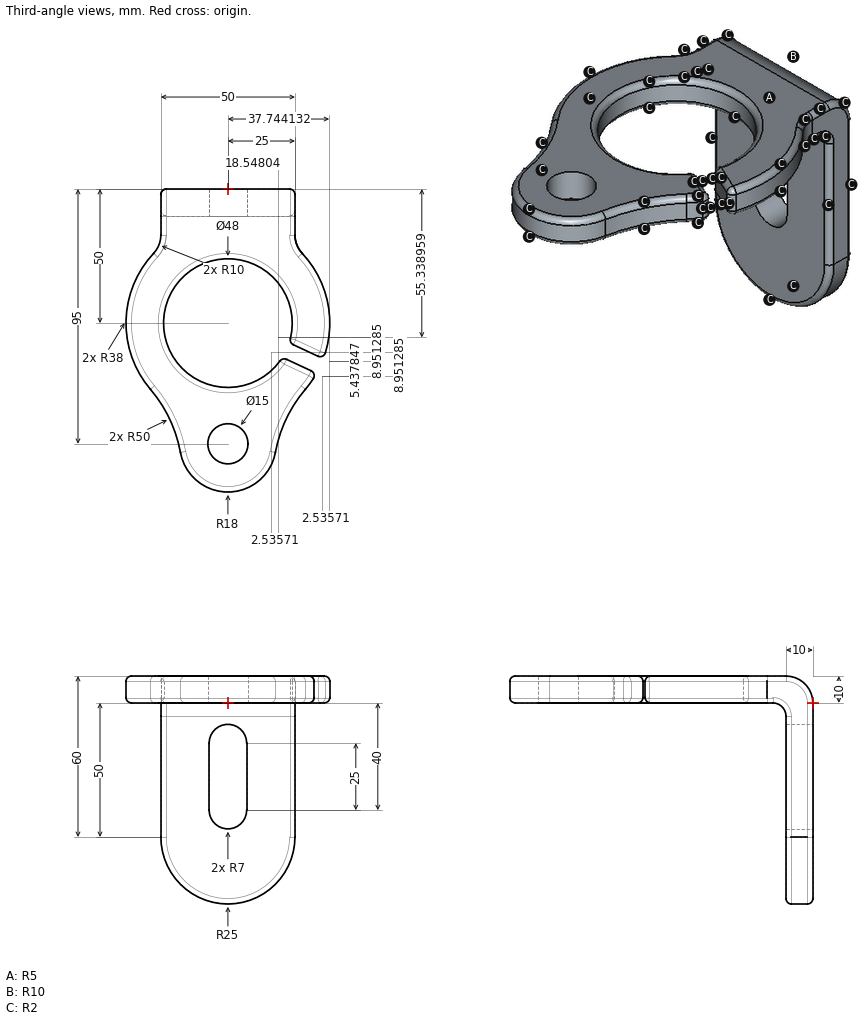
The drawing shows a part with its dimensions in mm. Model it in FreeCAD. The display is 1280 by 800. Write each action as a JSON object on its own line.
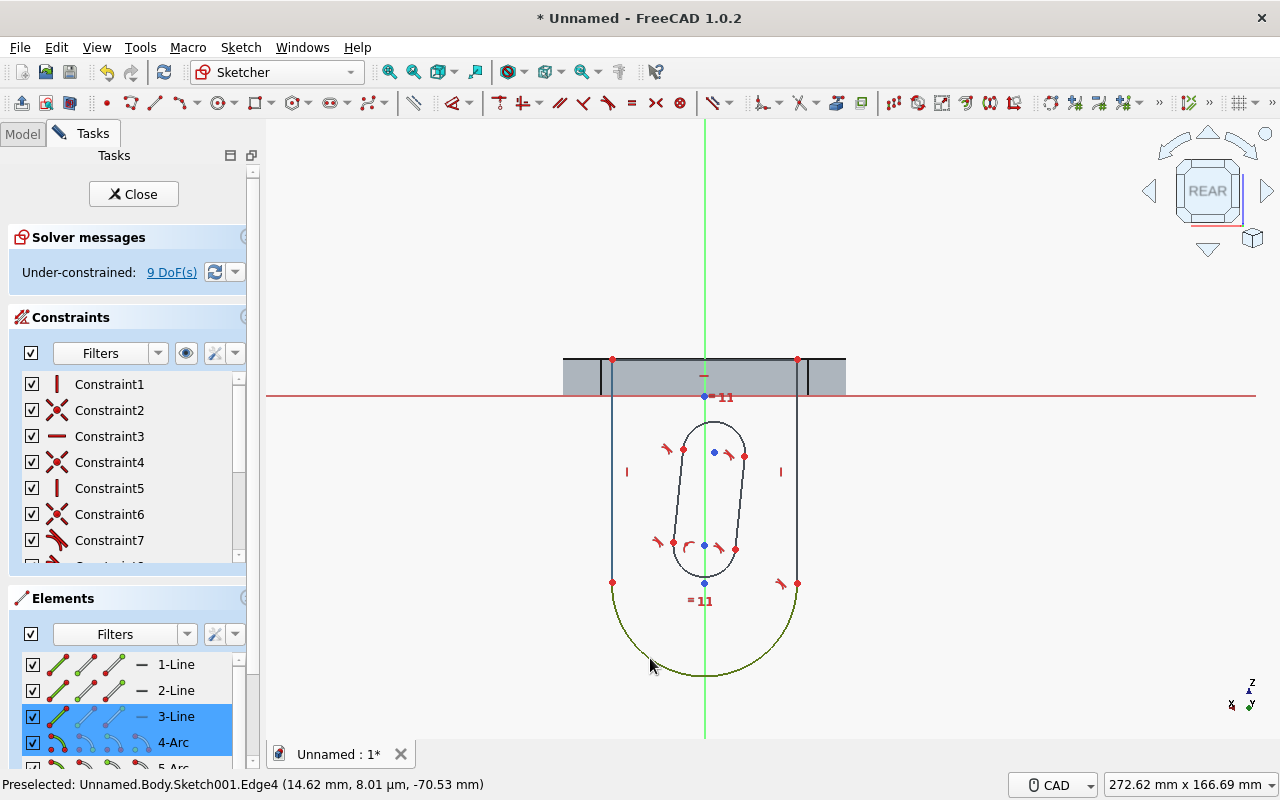
{"action": "left_click", "coordinate": [608, 104]}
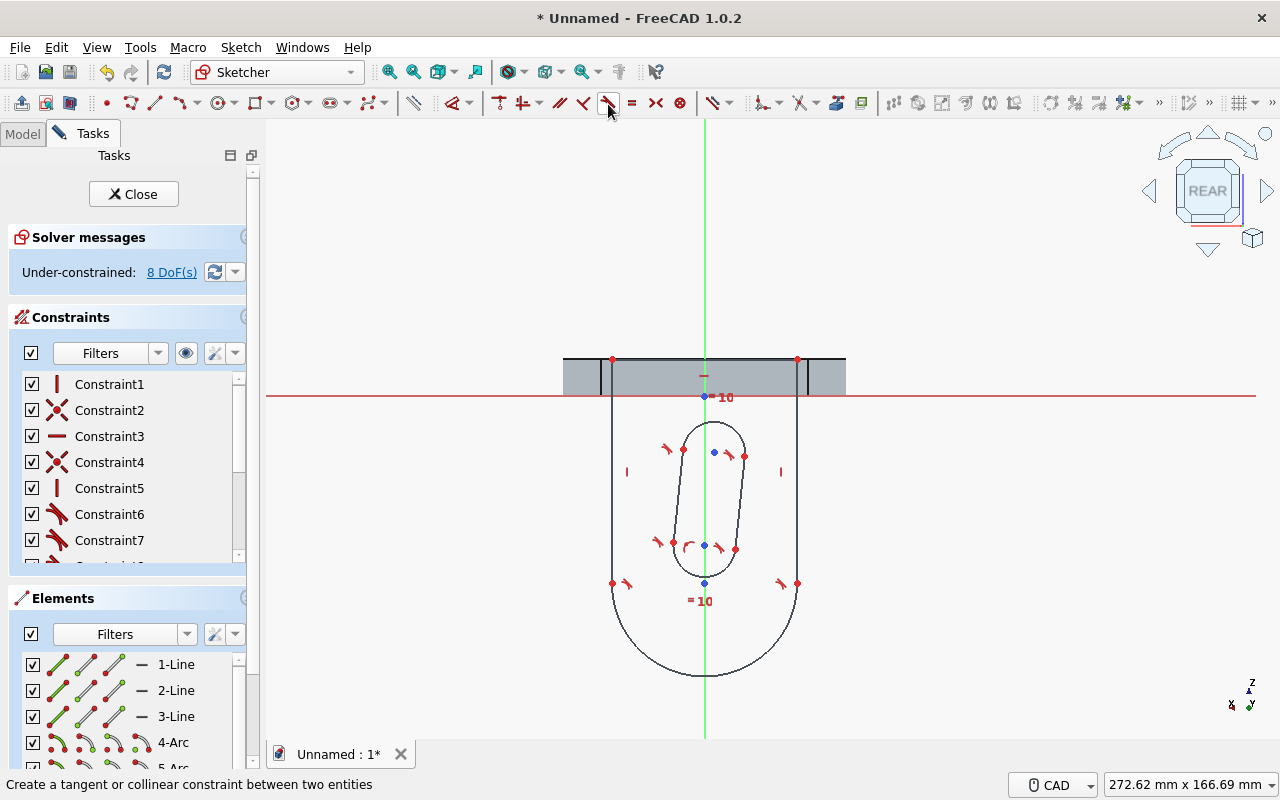
{"action": "left_click", "coordinate": [676, 515]}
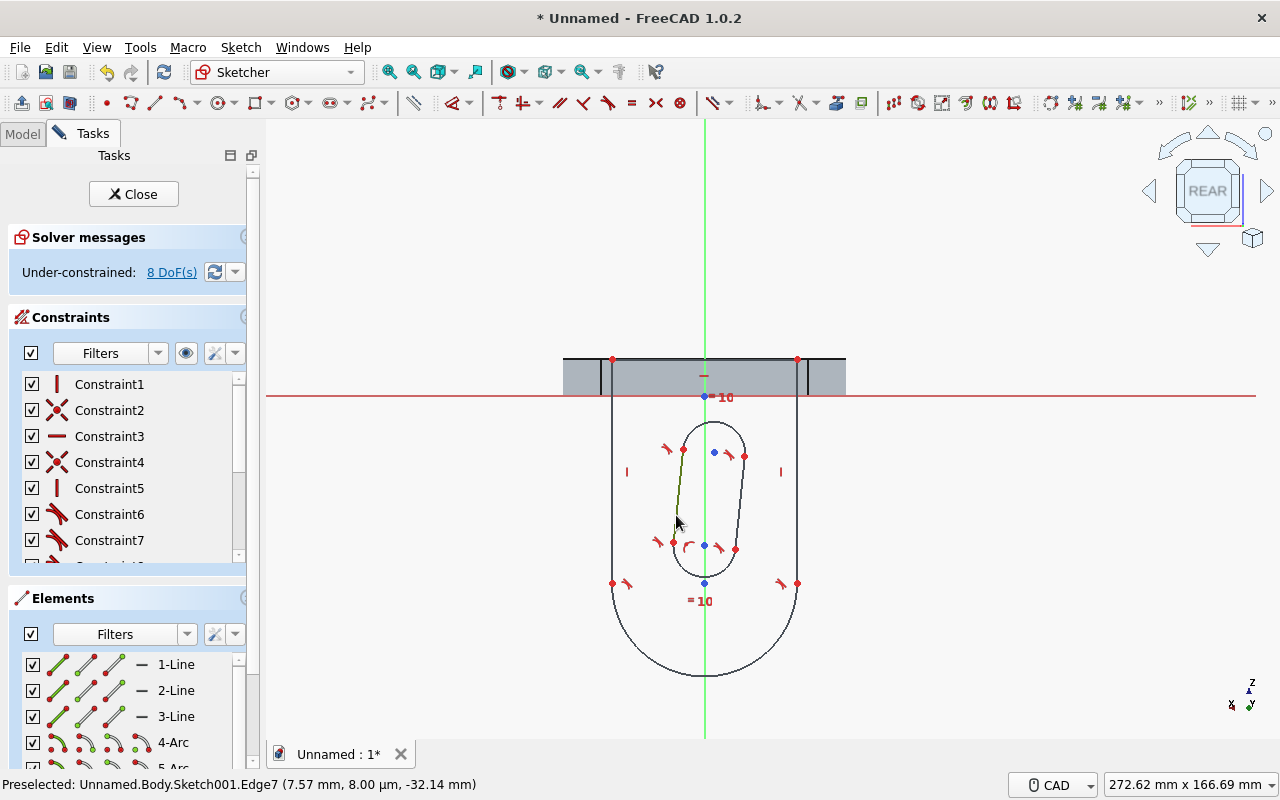
{"action": "key", "text": "v"}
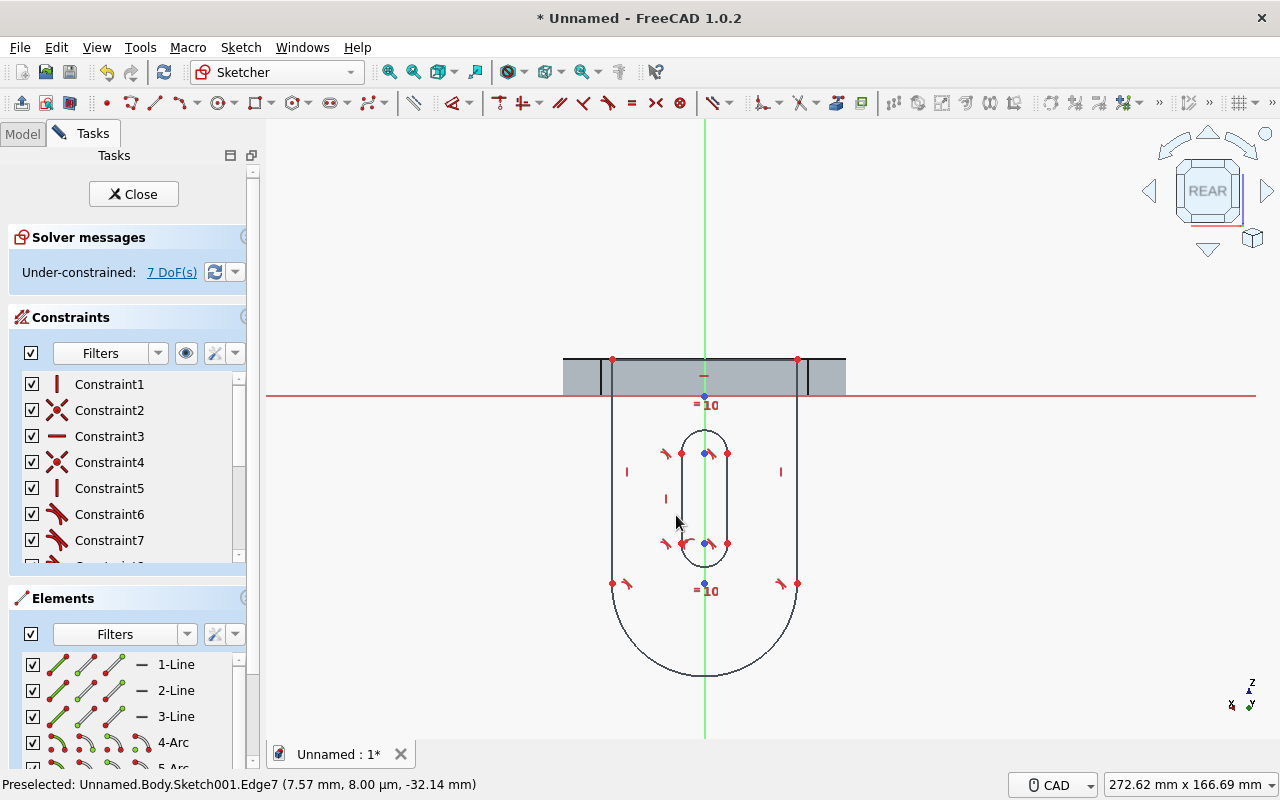
{"action": "left_click", "coordinate": [705, 584]}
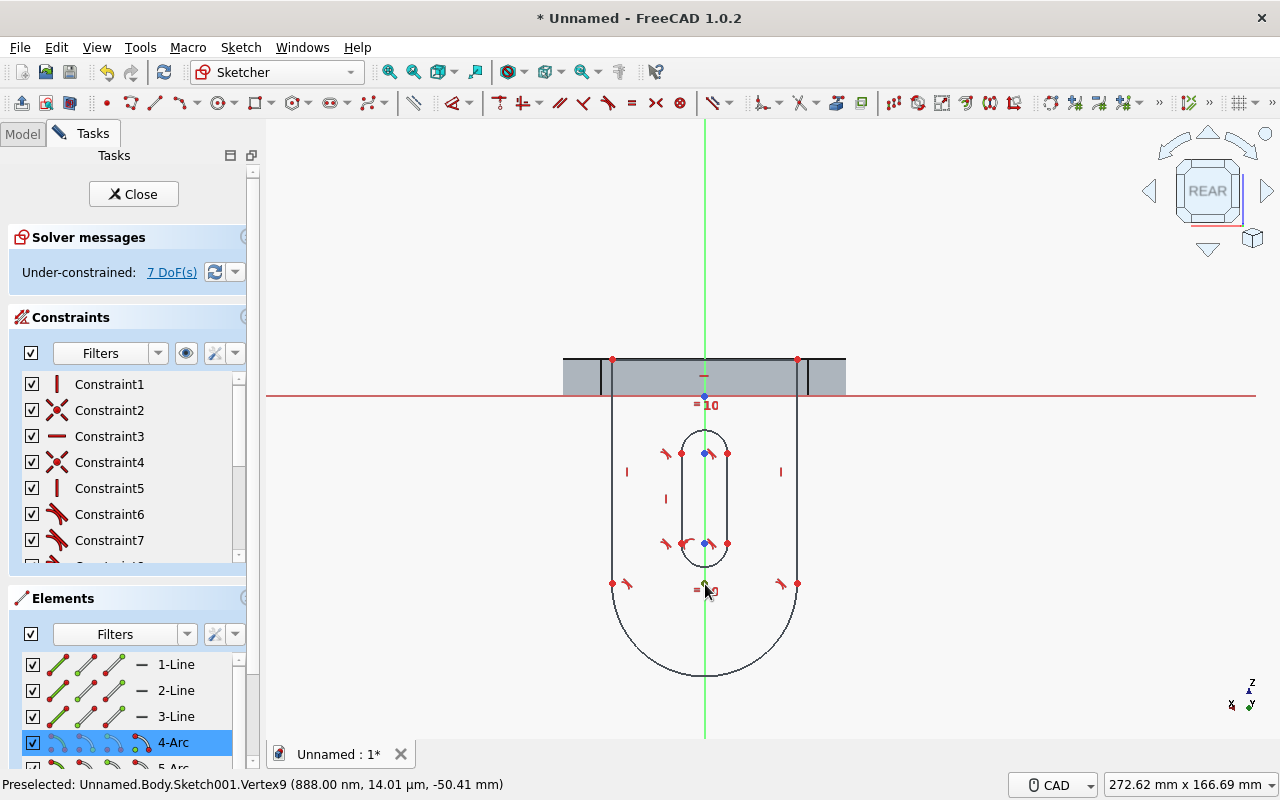
{"action": "left_click", "coordinate": [705, 630]}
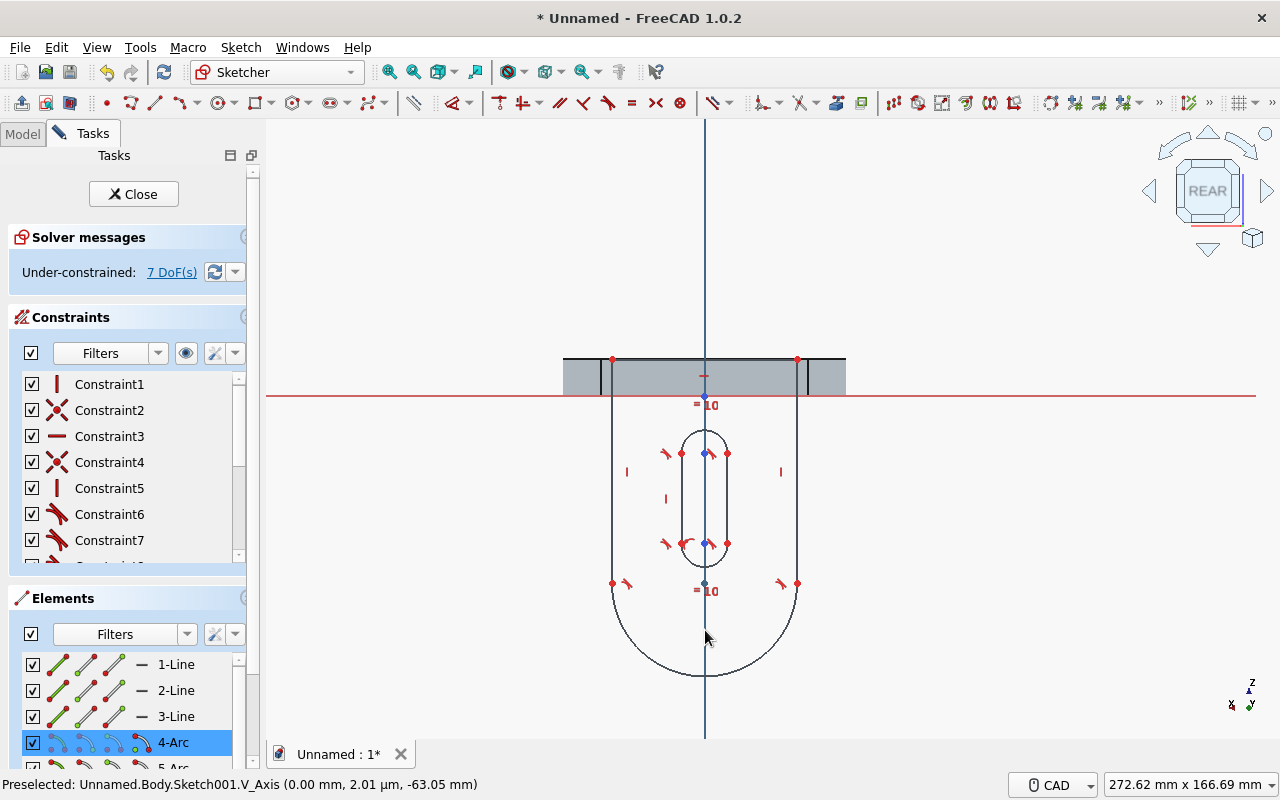
{"action": "left_click", "coordinate": [500, 104]}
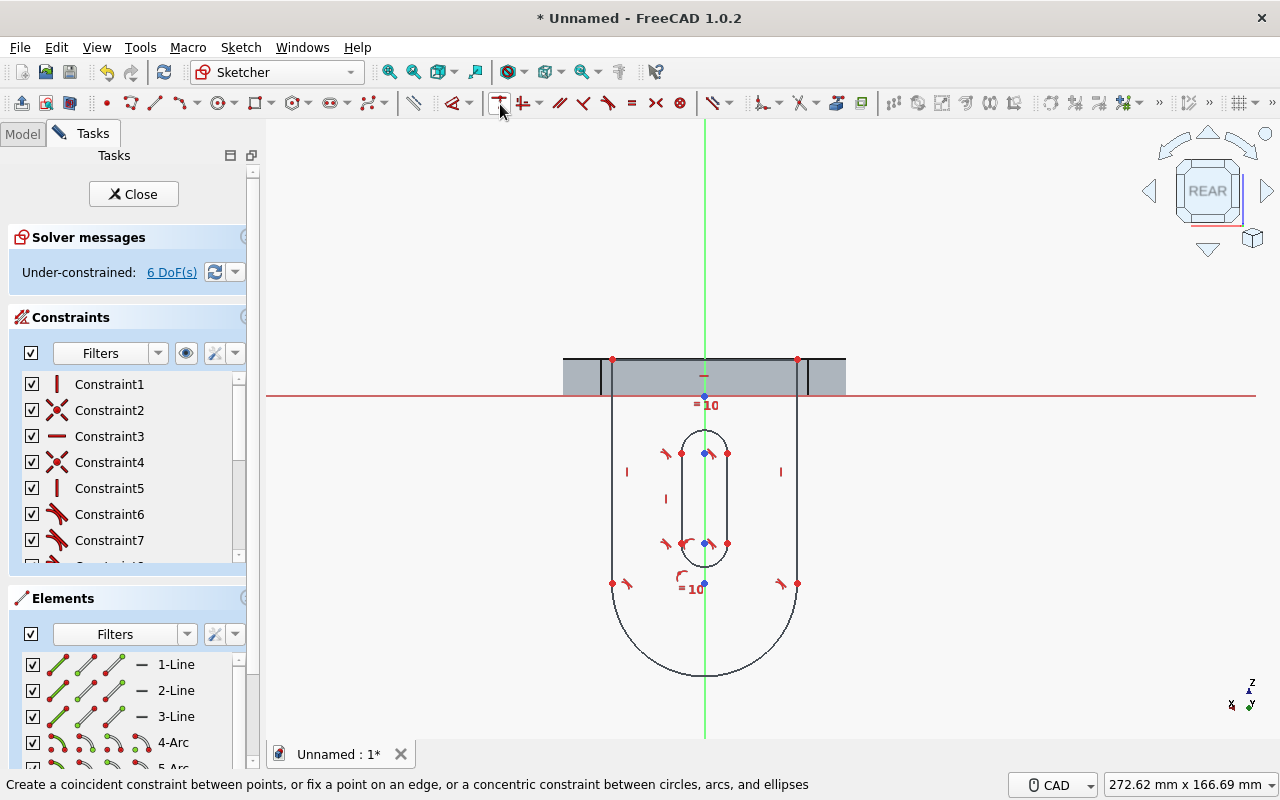
{"action": "left_click", "coordinate": [452, 104]}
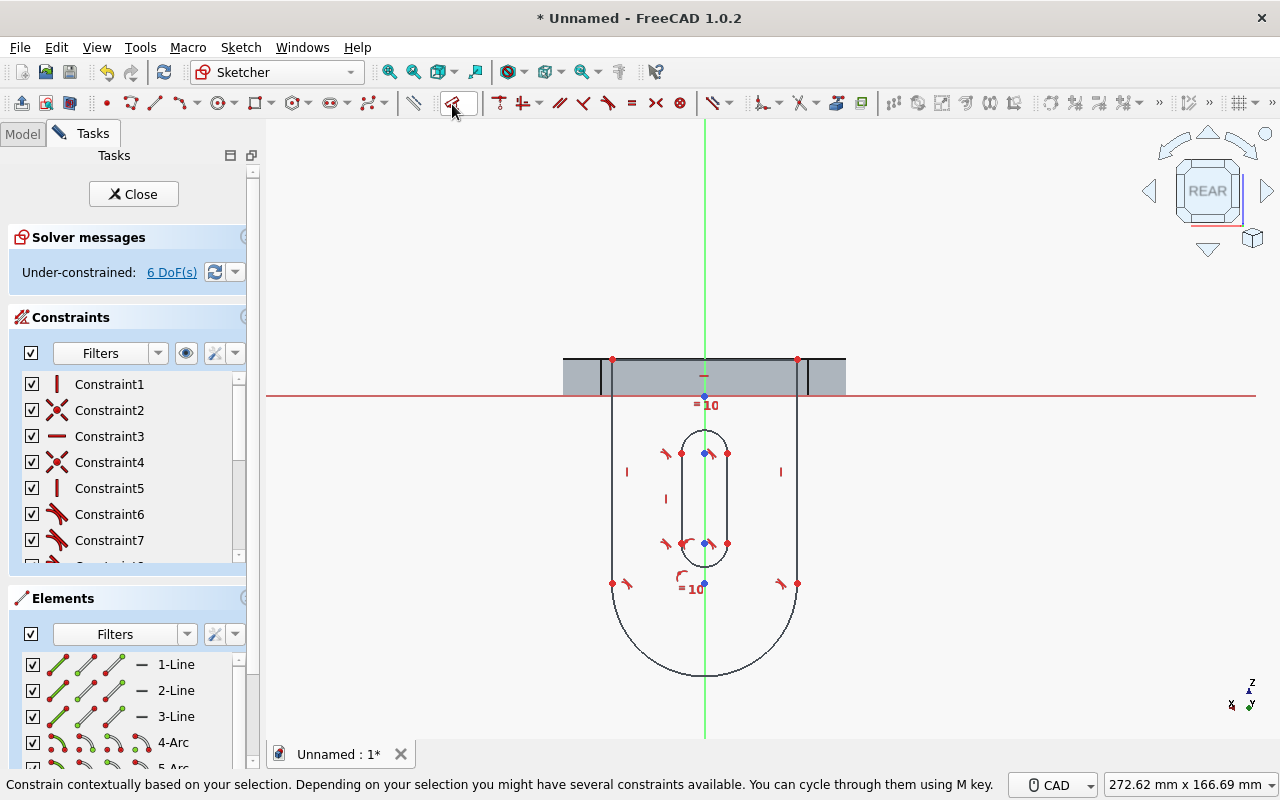
{"action": "left_click", "coordinate": [650, 659]}
{"action": "left_click", "coordinate": [631, 685]}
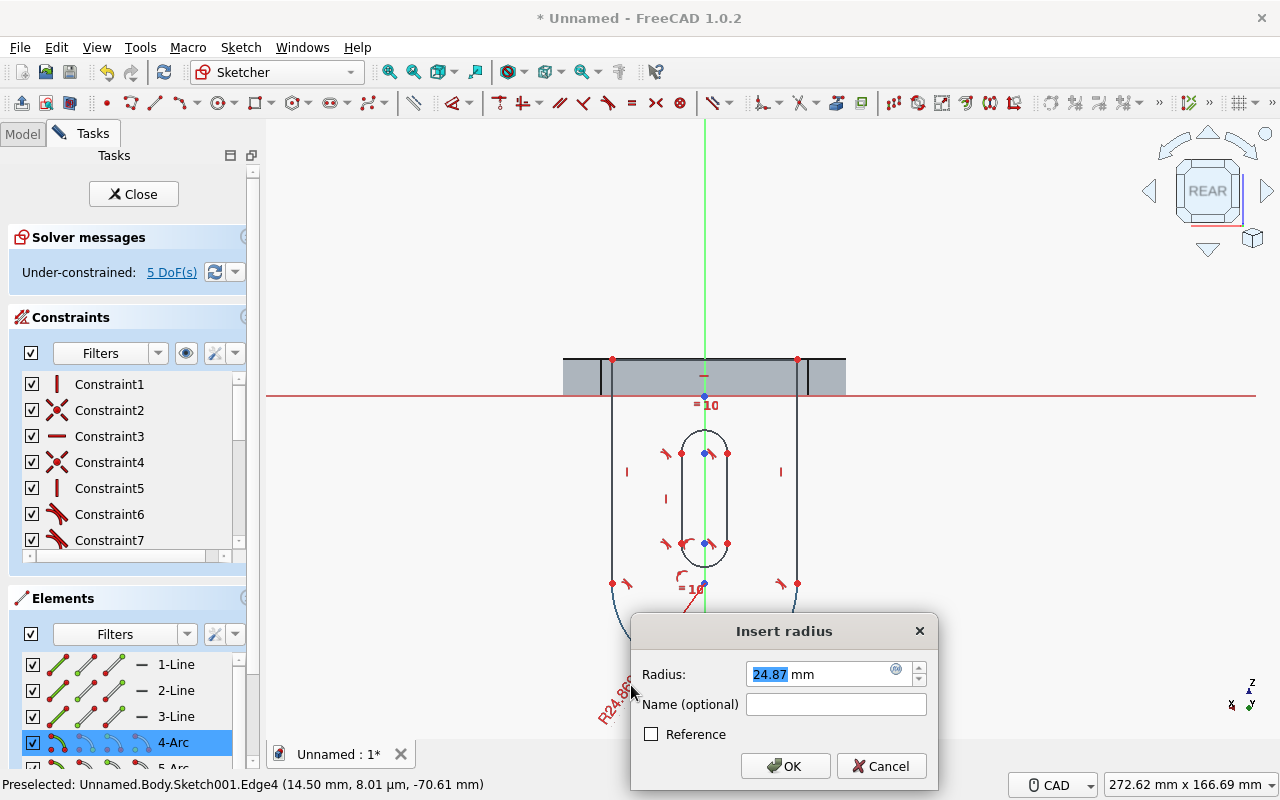
{"action": "type", "text": "25"}
{"action": "key", "text": "Return"}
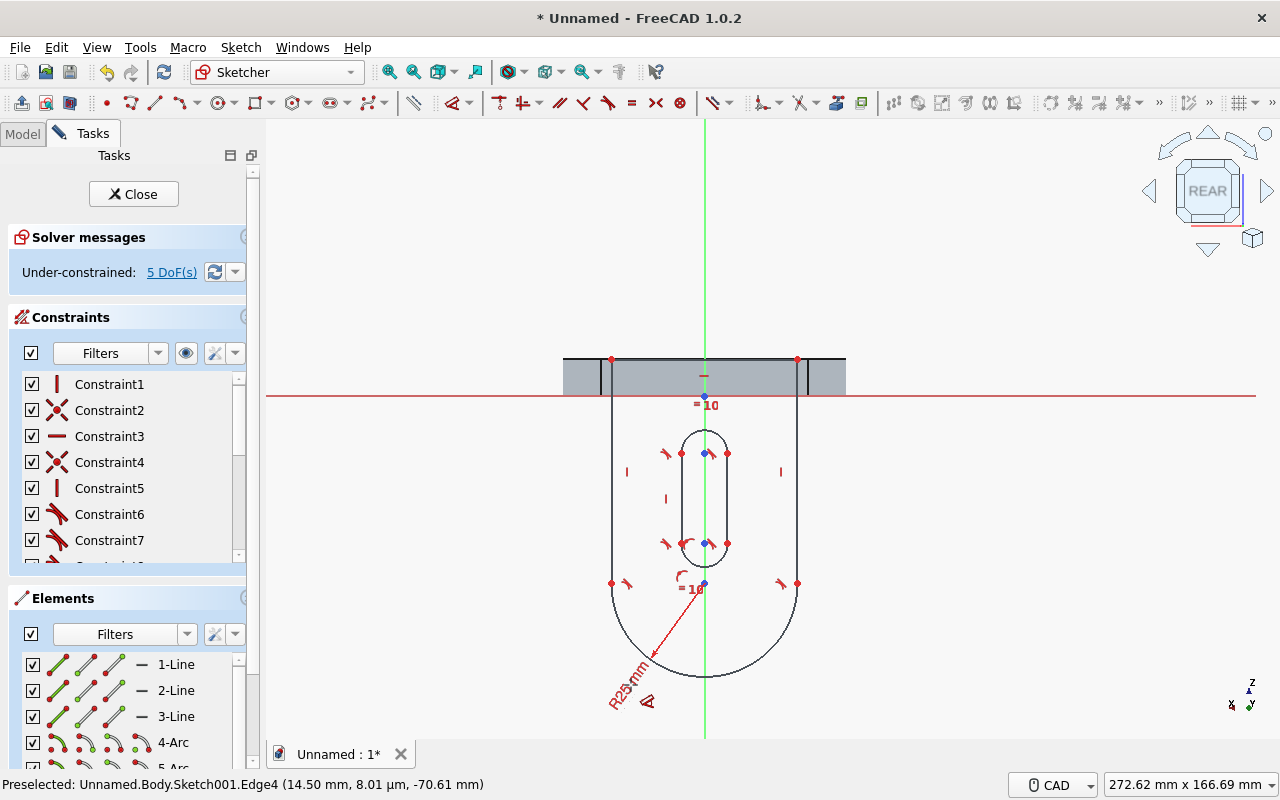
{"action": "scroll", "coordinate": [691, 563], "scroll_direction": "up", "scroll_amount": 3}